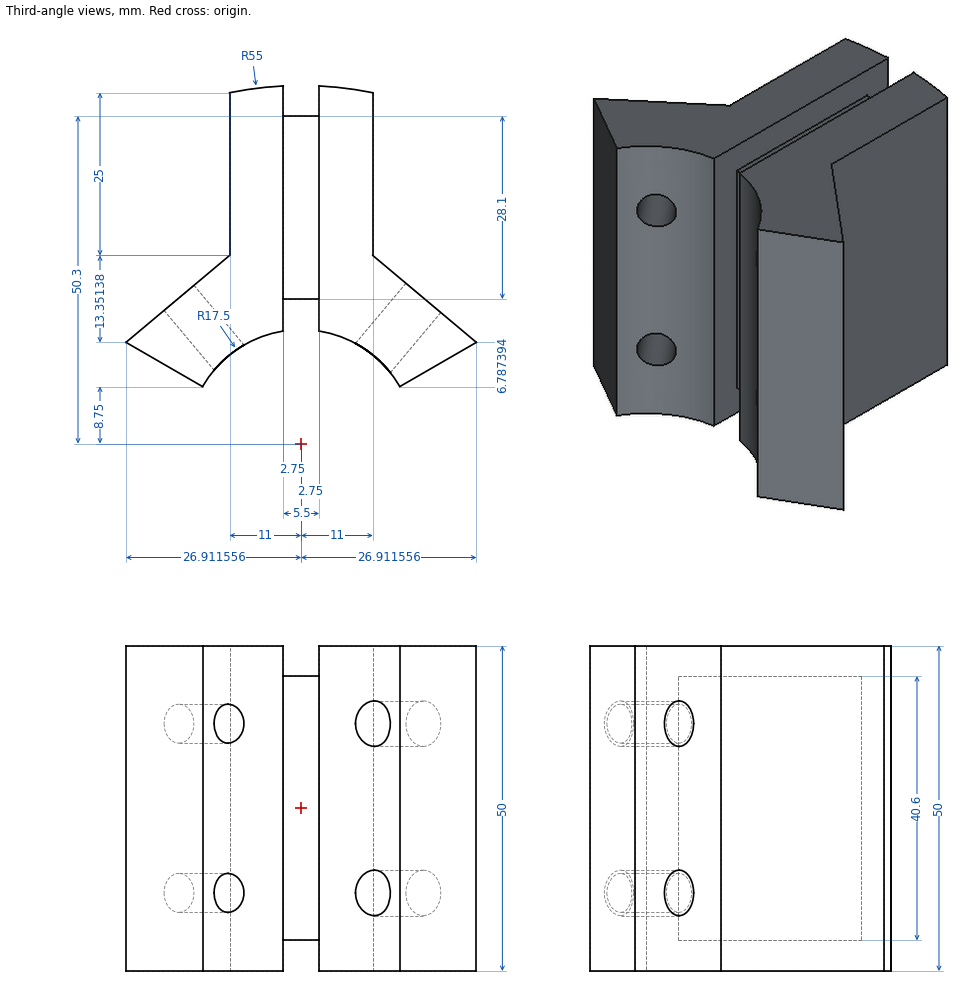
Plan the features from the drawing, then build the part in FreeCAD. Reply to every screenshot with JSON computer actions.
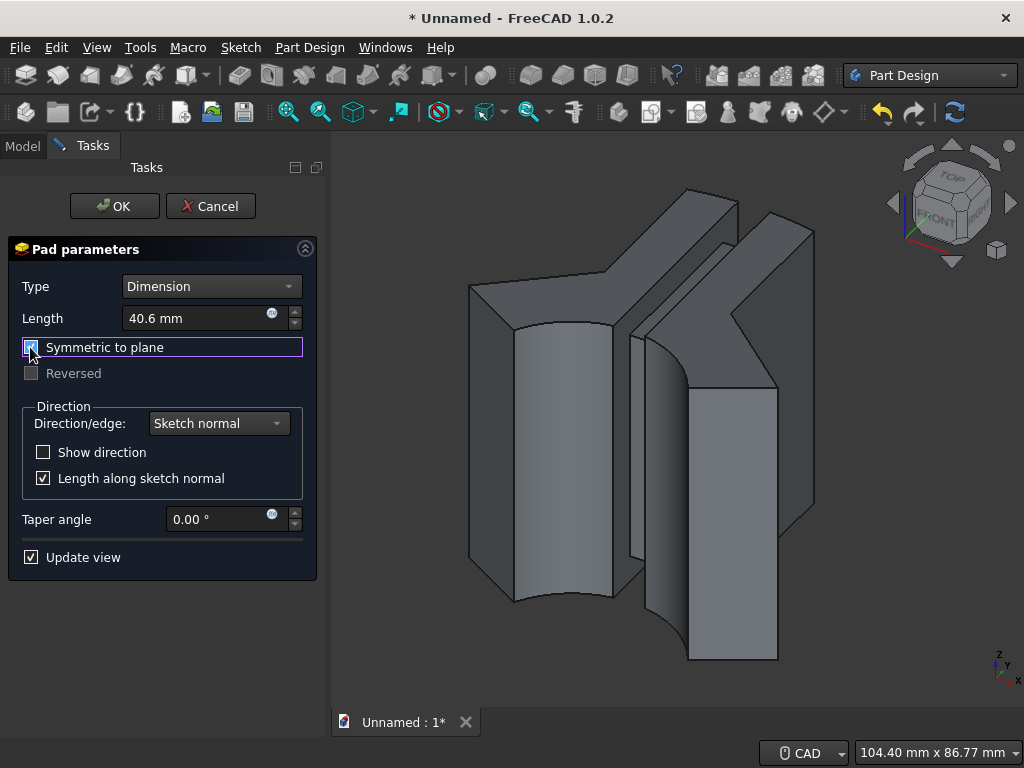
{"action": "left_click", "coordinate": [115, 206]}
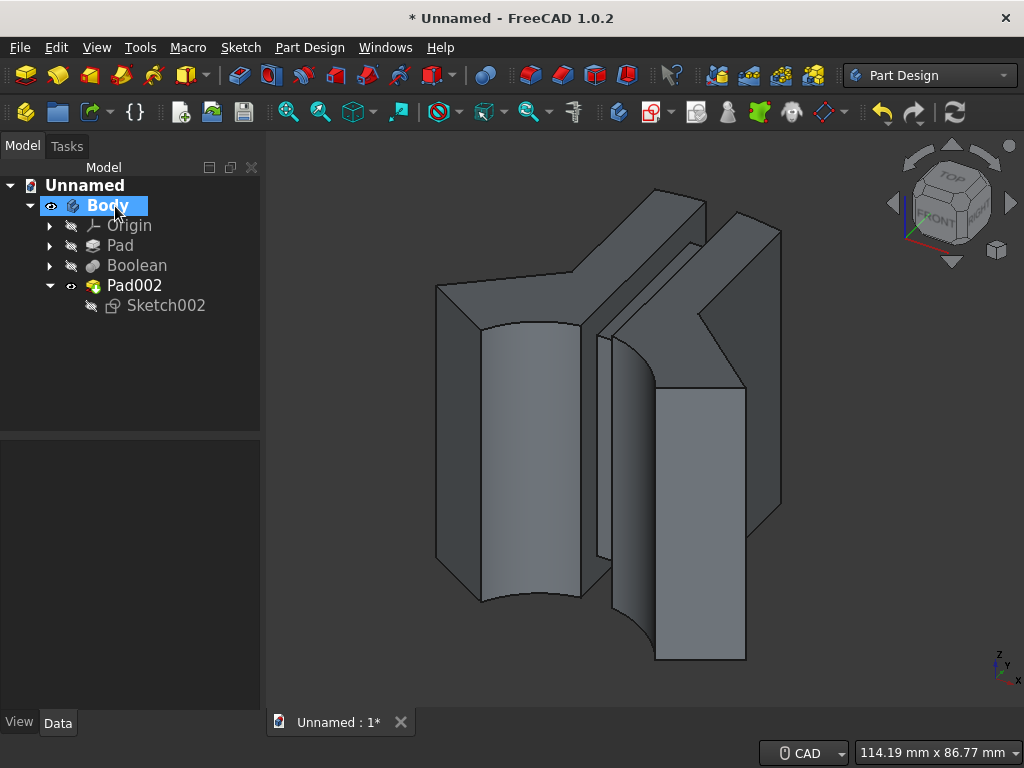
{"action": "key", "text": "4"}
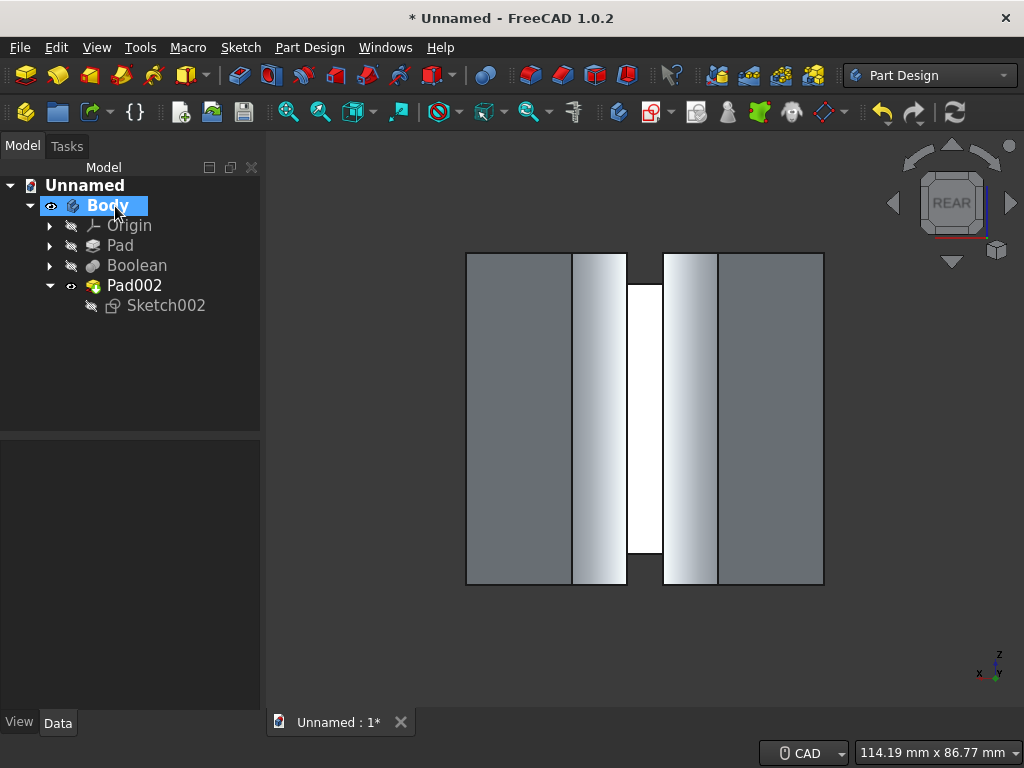
{"action": "left_click", "coordinate": [771, 323]}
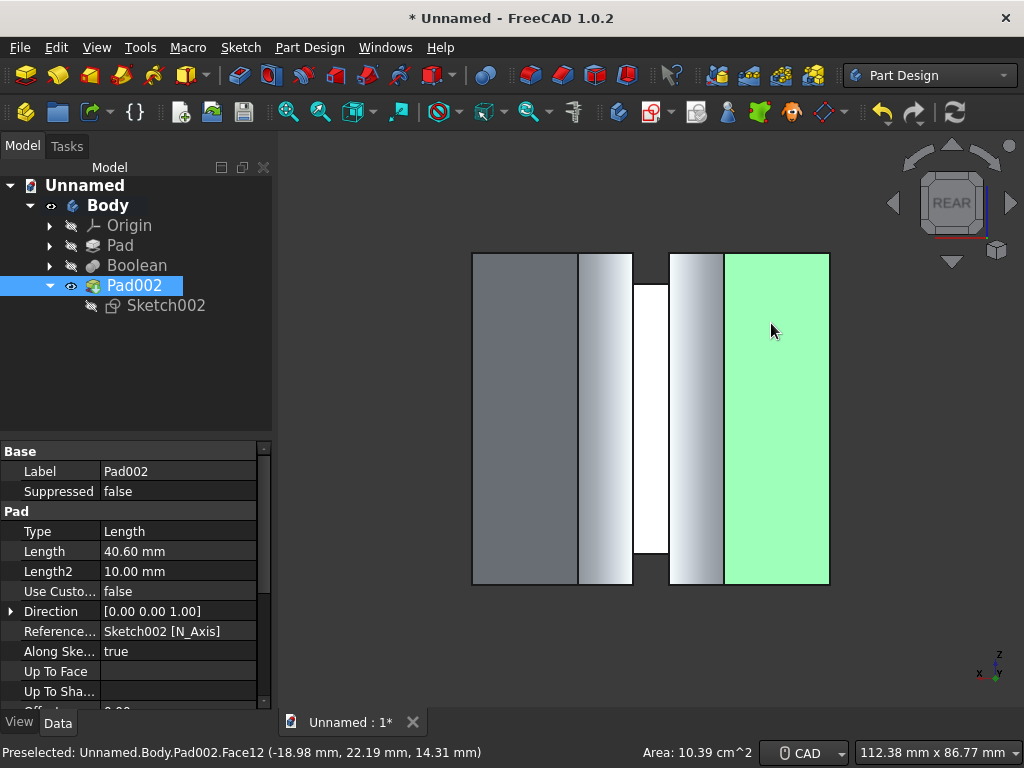
{"action": "left_click", "coordinate": [652, 112]}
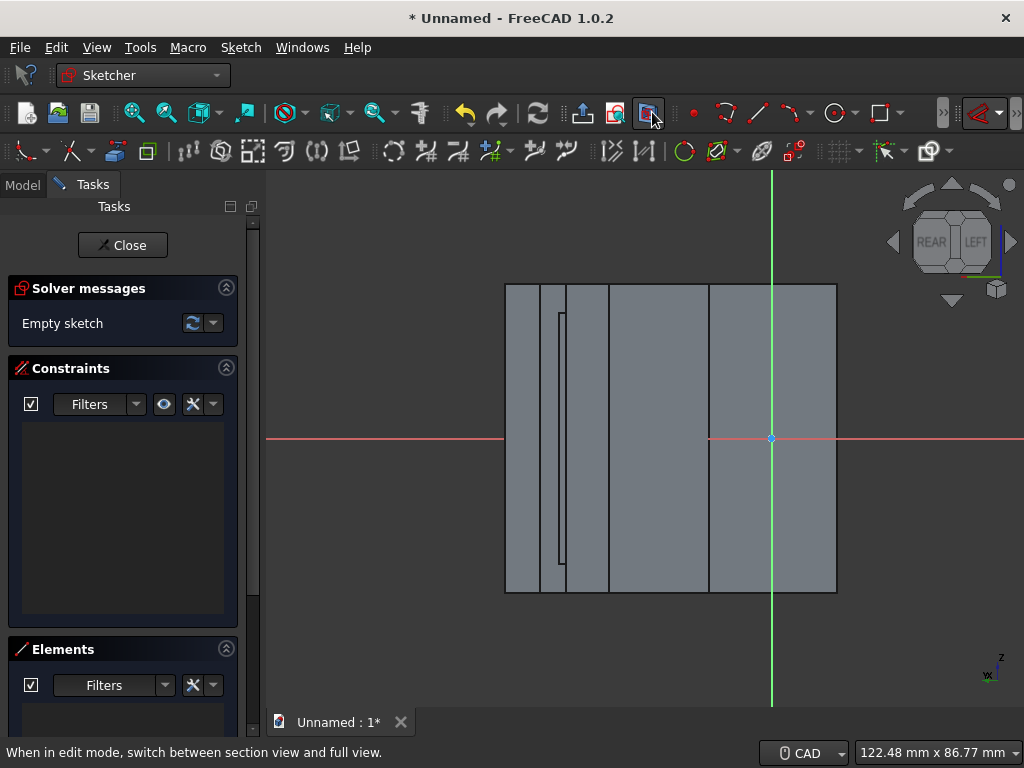
{"action": "left_click", "coordinate": [648, 114]}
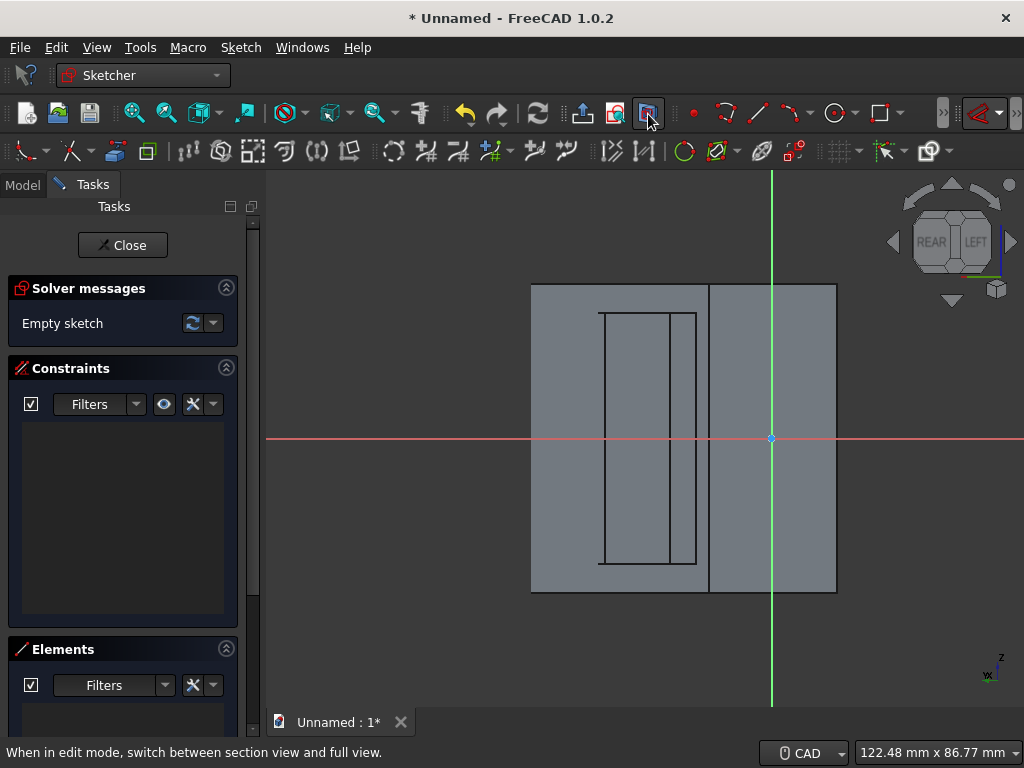
{"action": "scroll", "coordinate": [796, 348], "scroll_direction": "up", "scroll_amount": 11}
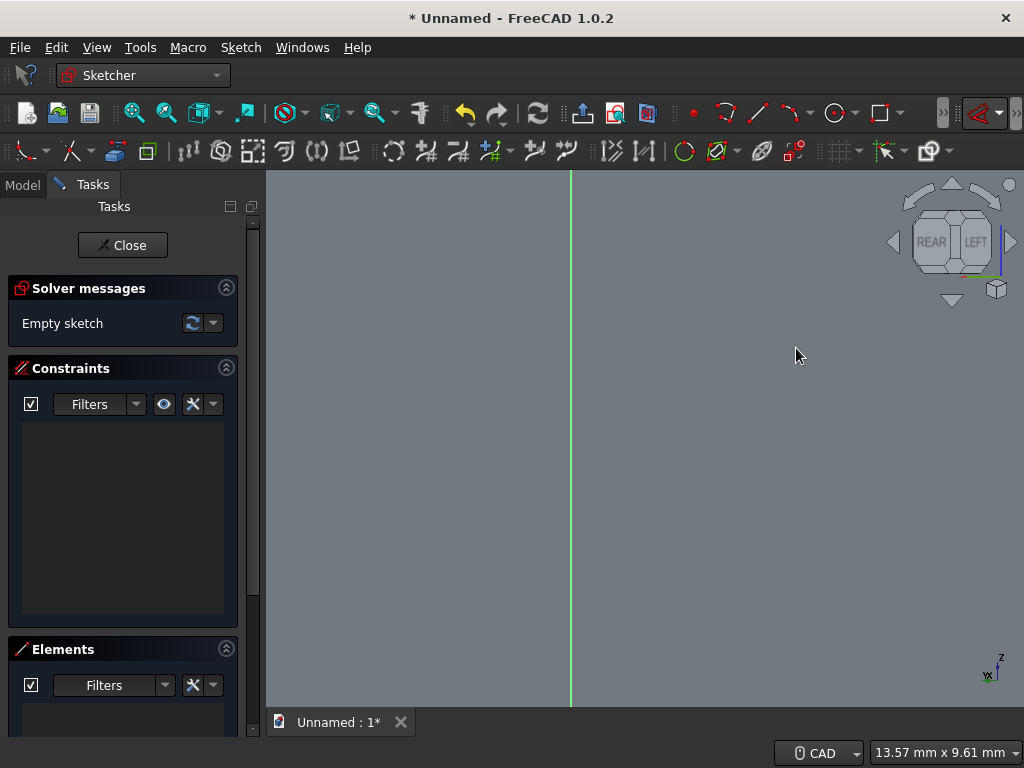
{"action": "left_click", "coordinate": [836, 114]}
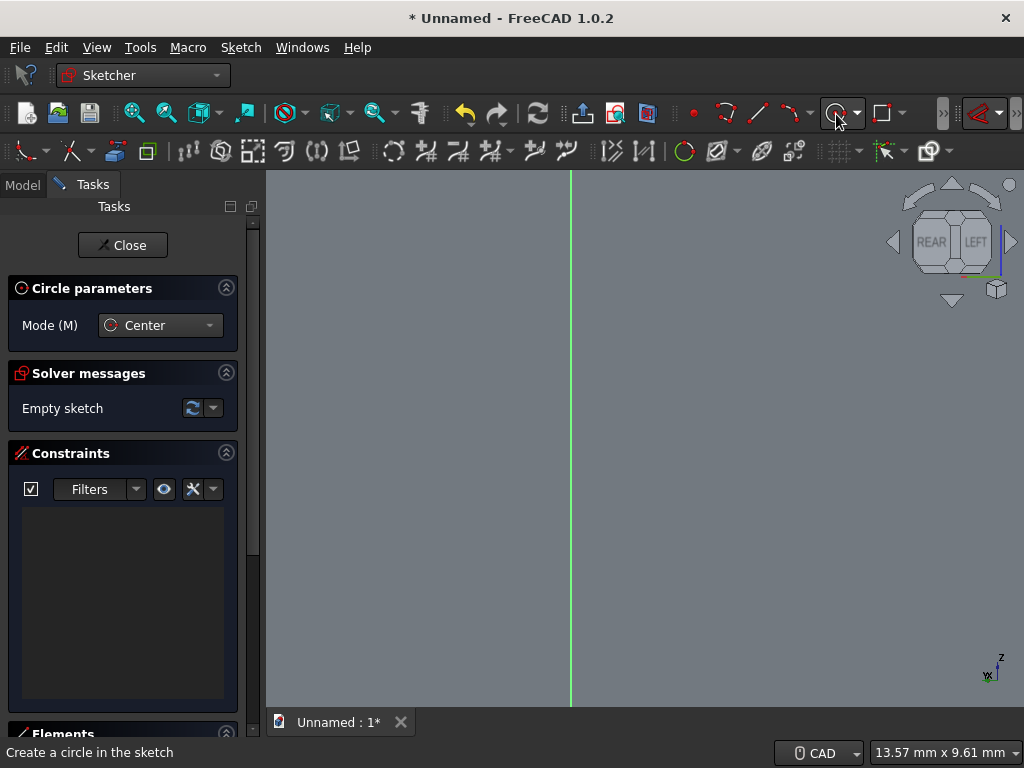
{"action": "left_click", "coordinate": [571, 436]}
{"action": "mouse_move", "coordinate": [689, 318]}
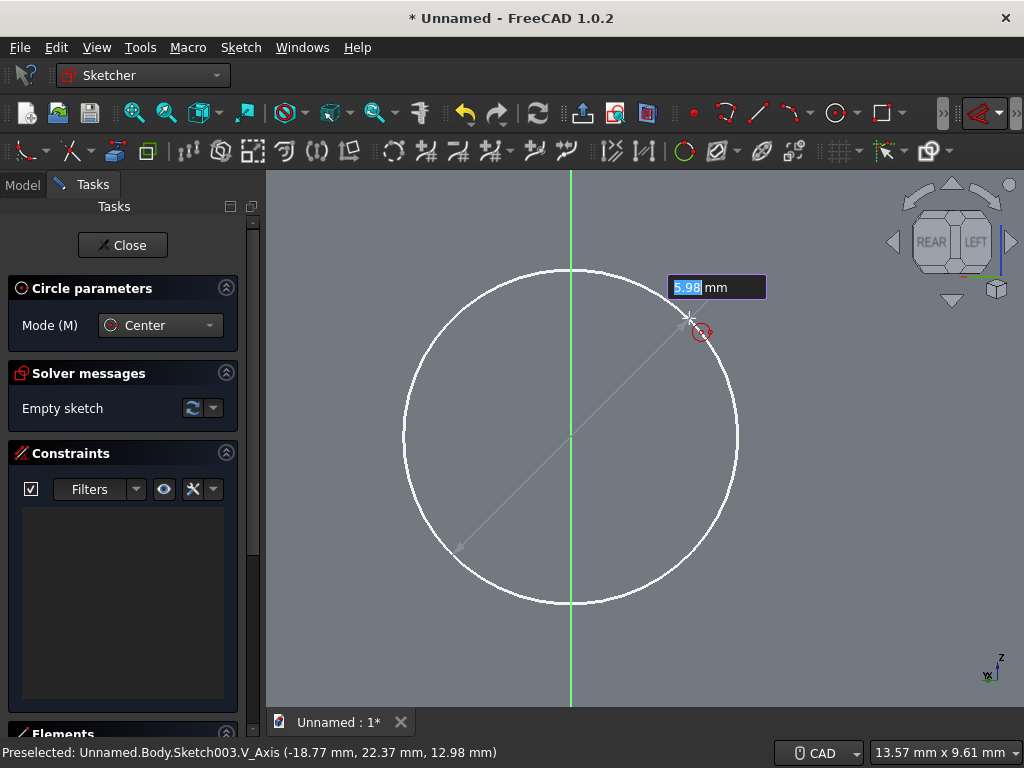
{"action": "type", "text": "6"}
{"action": "key", "text": "Return"}
{"action": "key", "text": "Escape"}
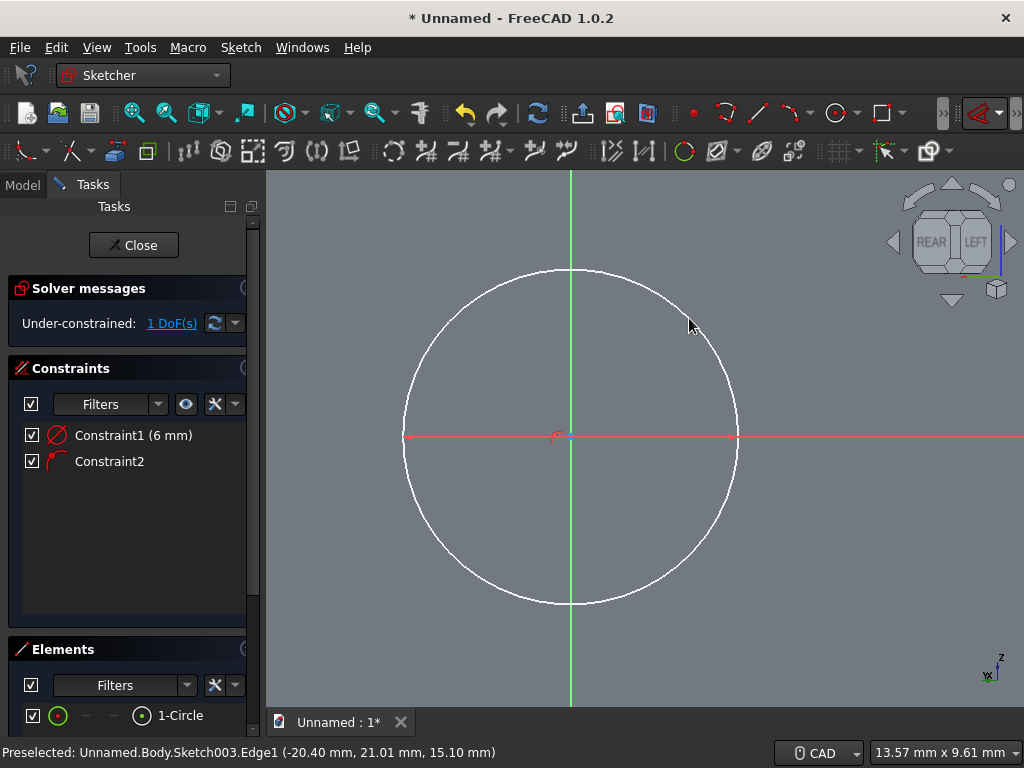
{"action": "left_click", "coordinate": [571, 437]}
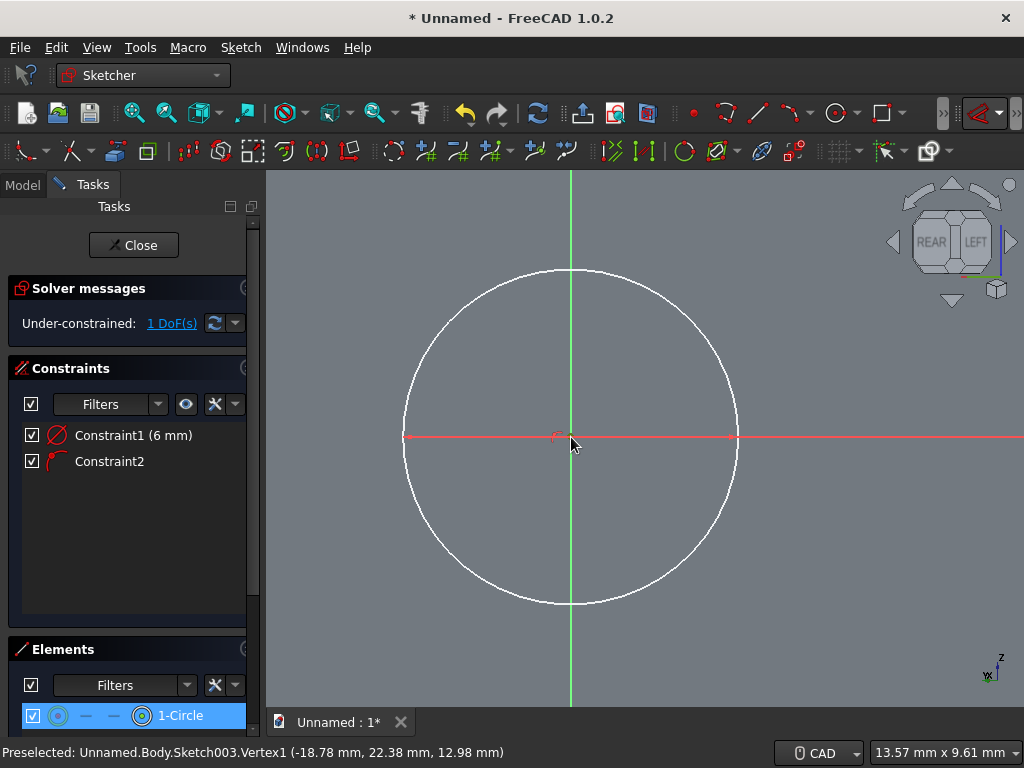
{"action": "left_click", "coordinate": [1002, 114]}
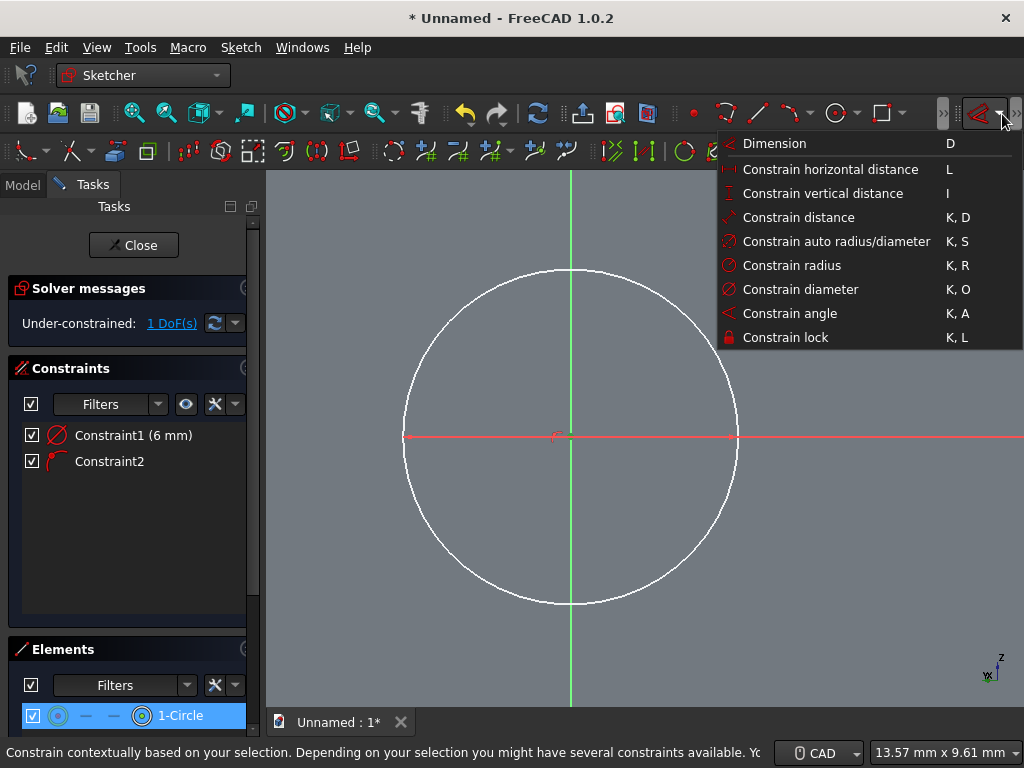
{"action": "left_click", "coordinate": [870, 193]}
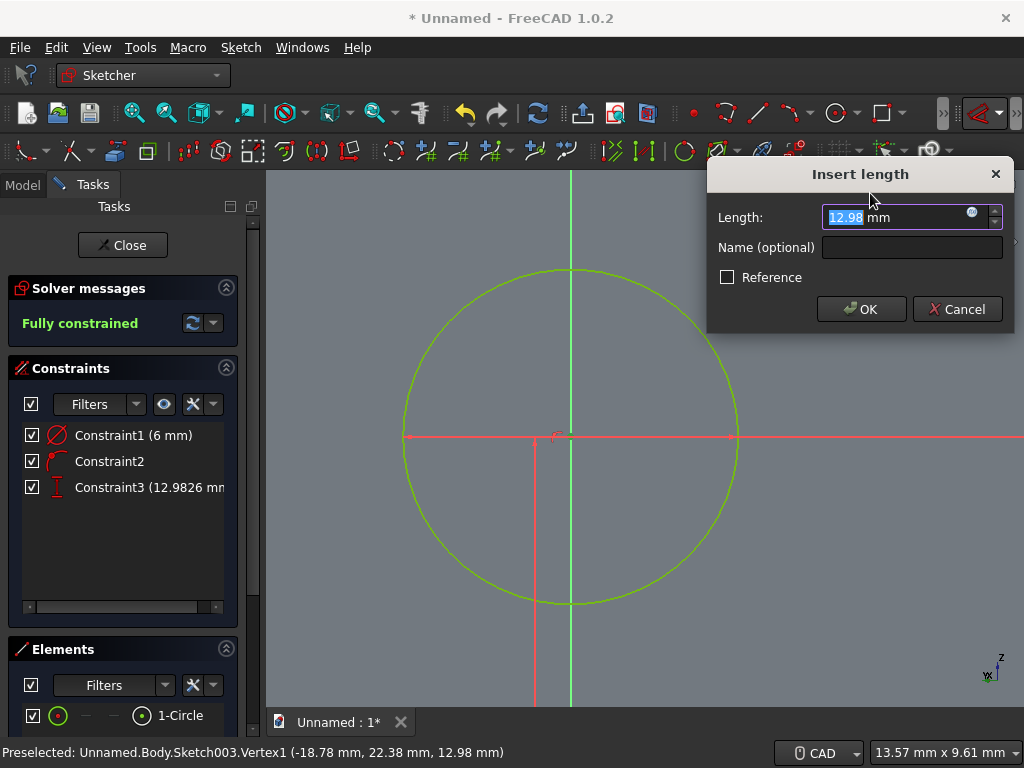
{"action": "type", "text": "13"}
{"action": "key", "text": "Return"}